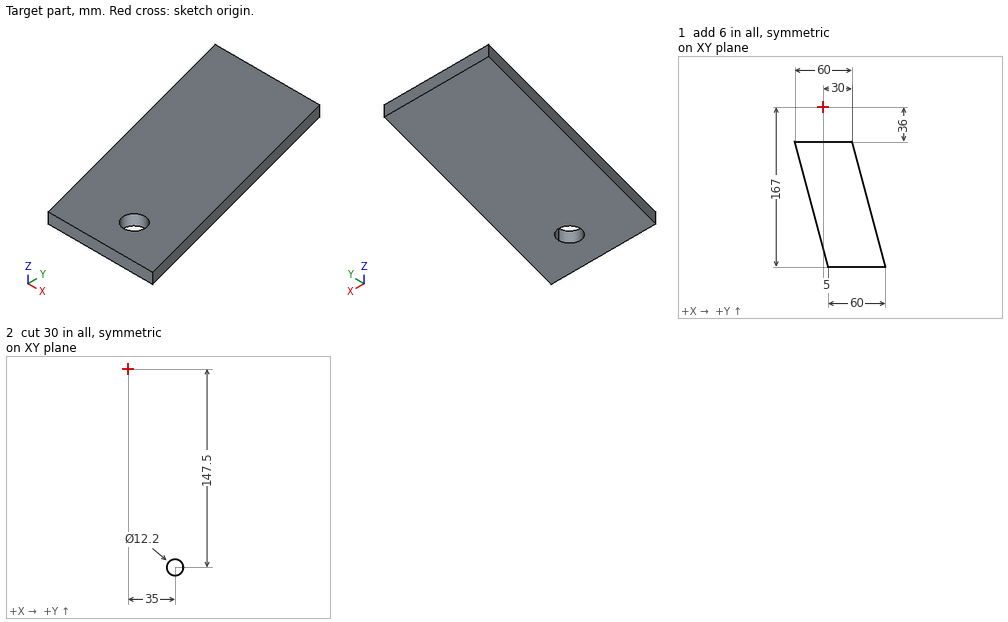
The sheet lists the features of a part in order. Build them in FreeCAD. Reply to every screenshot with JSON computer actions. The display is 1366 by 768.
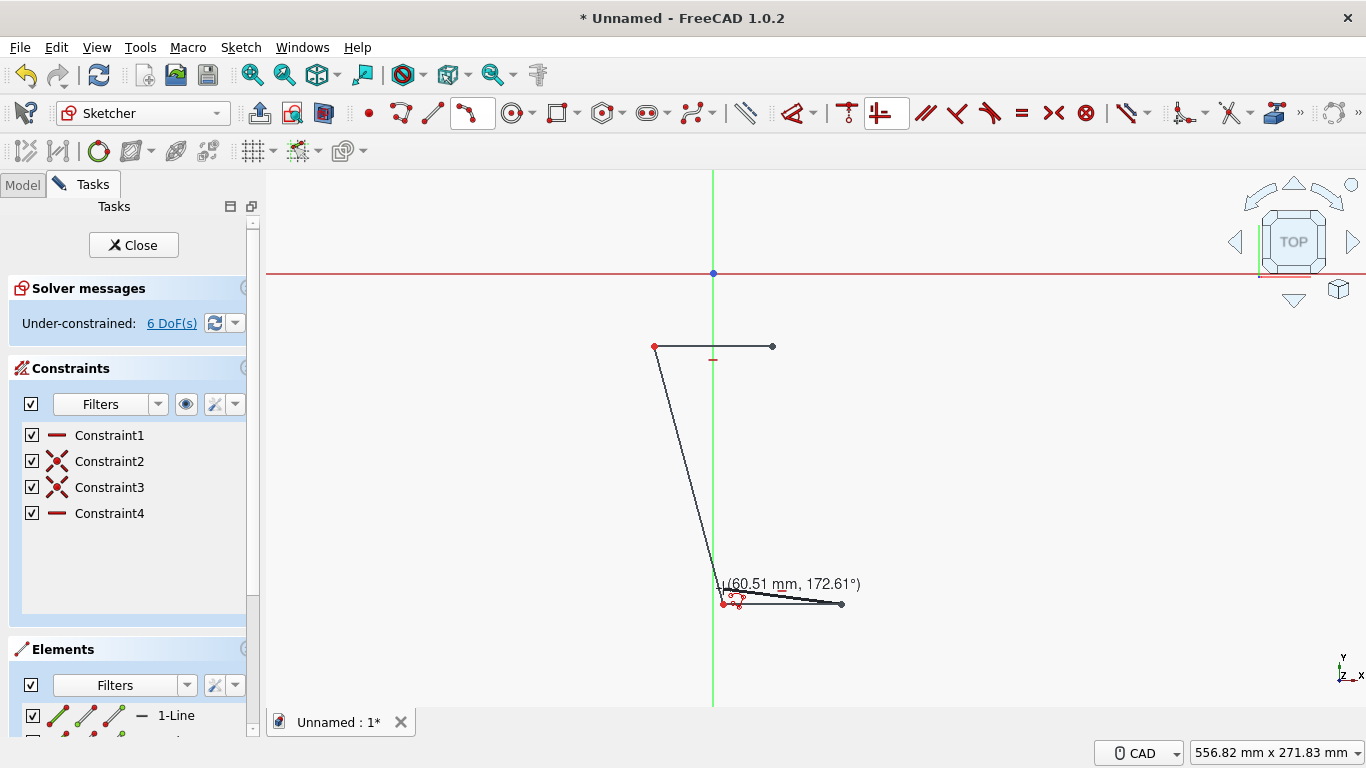
{"action": "left_click", "coordinate": [772, 346]}
{"action": "key", "text": "Escape"}
{"action": "key", "text": "Escape"}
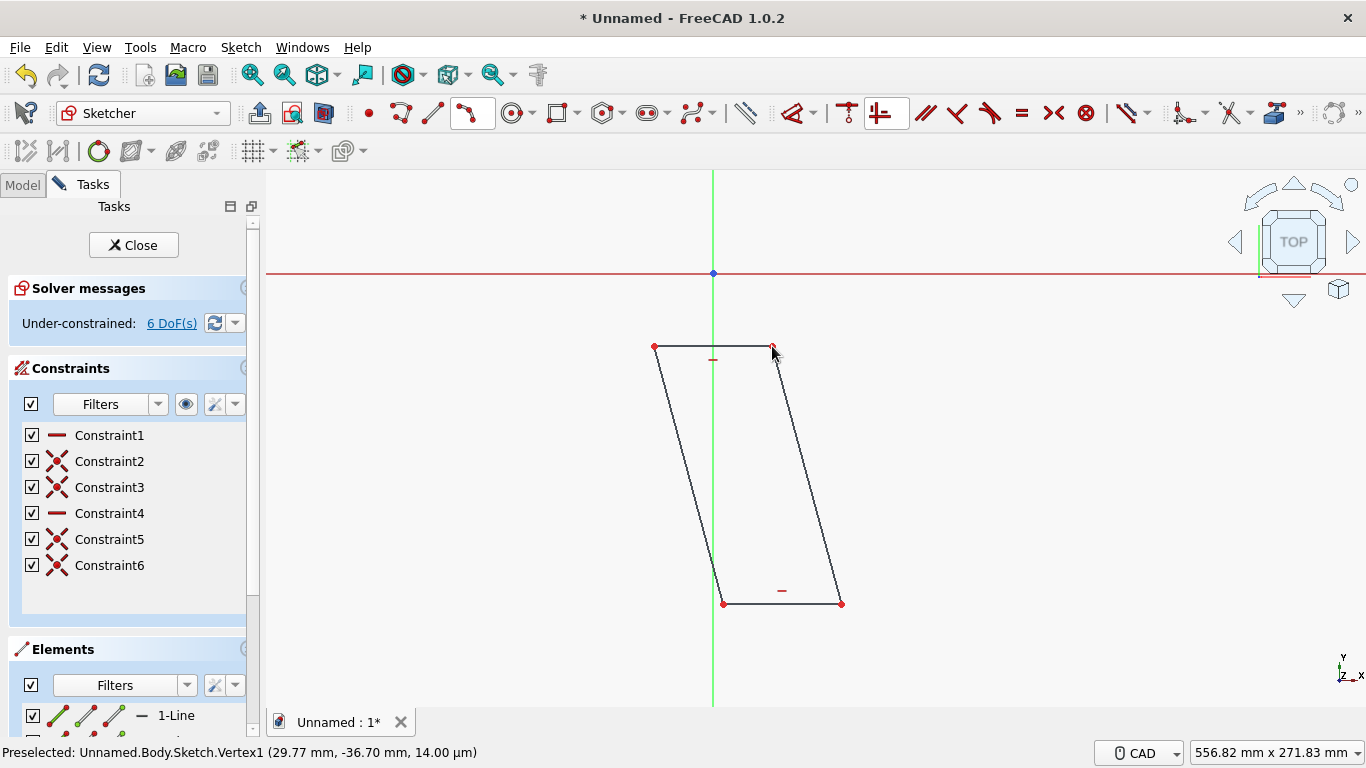
{"action": "left_click", "coordinate": [737, 346]}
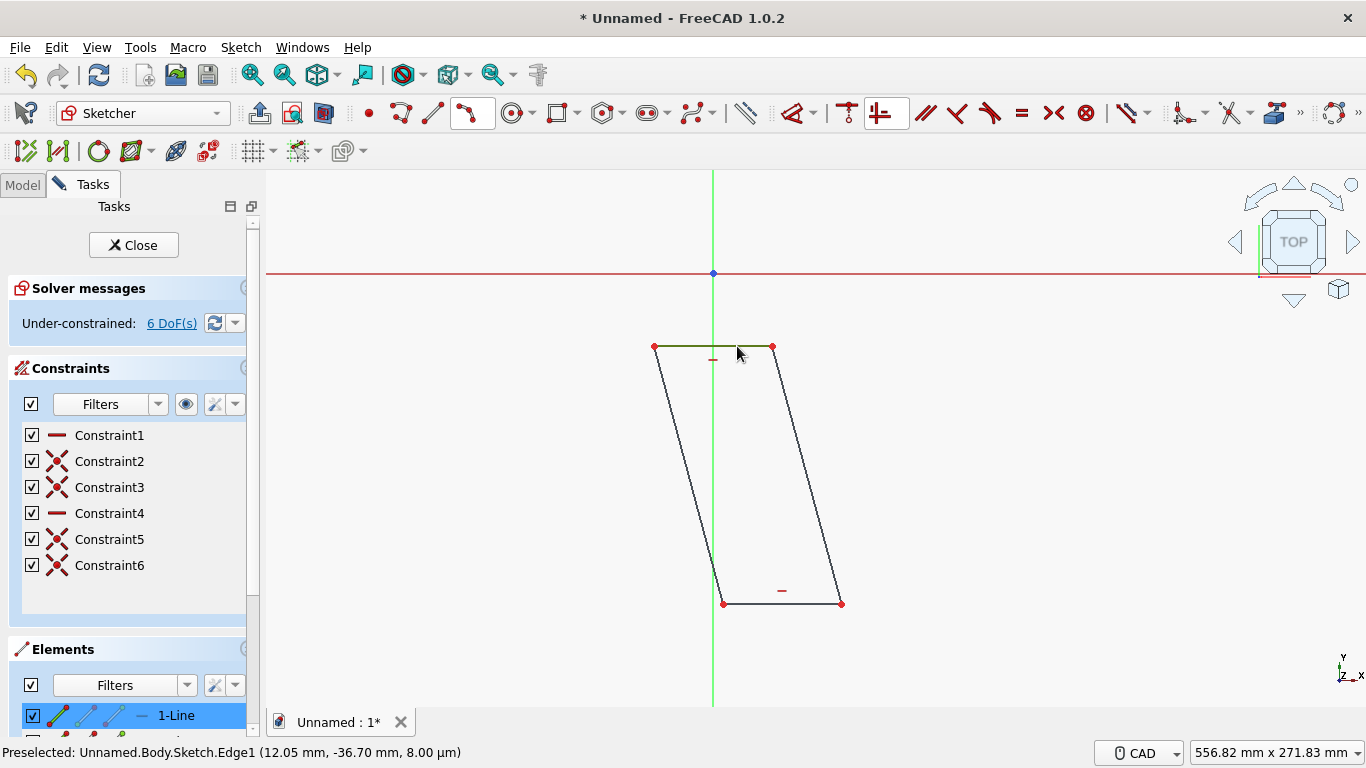
{"action": "left_click", "coordinate": [816, 114]}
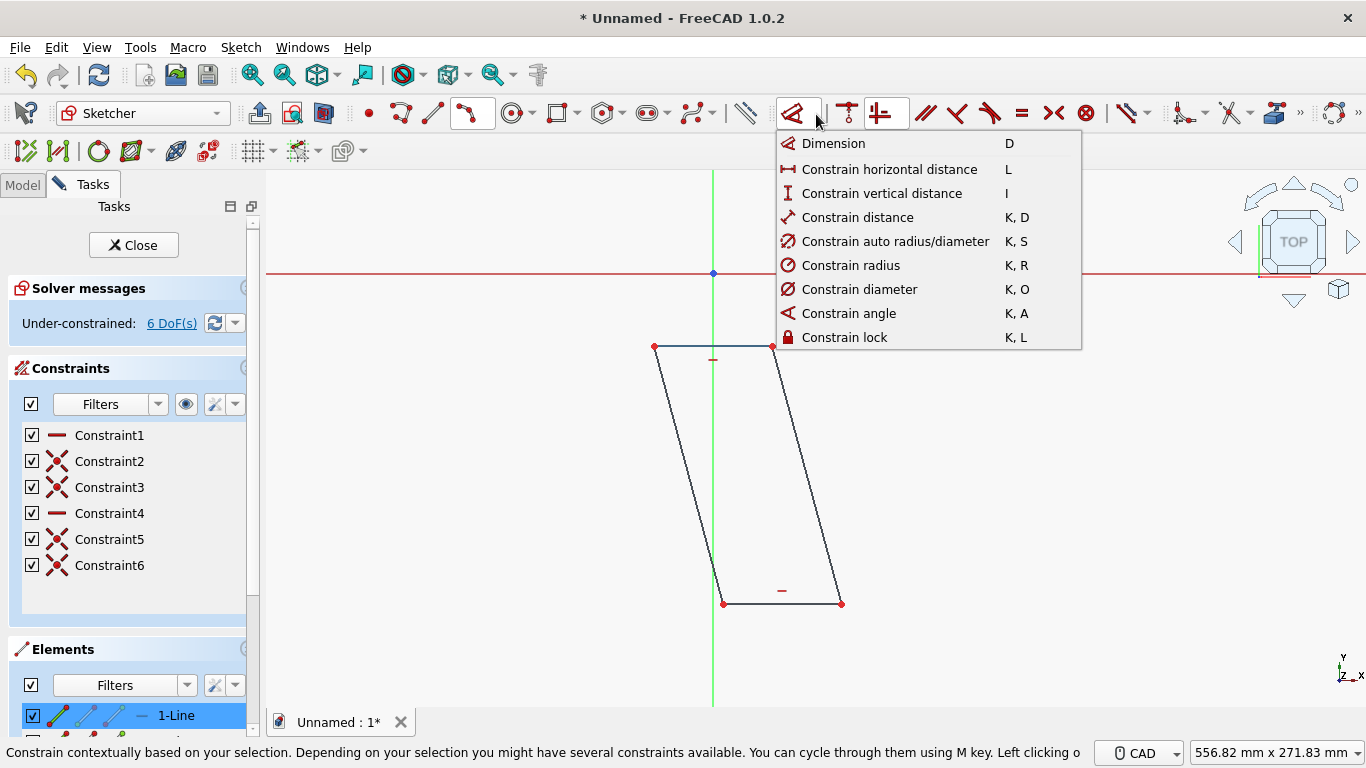
{"action": "left_click", "coordinate": [929, 169]}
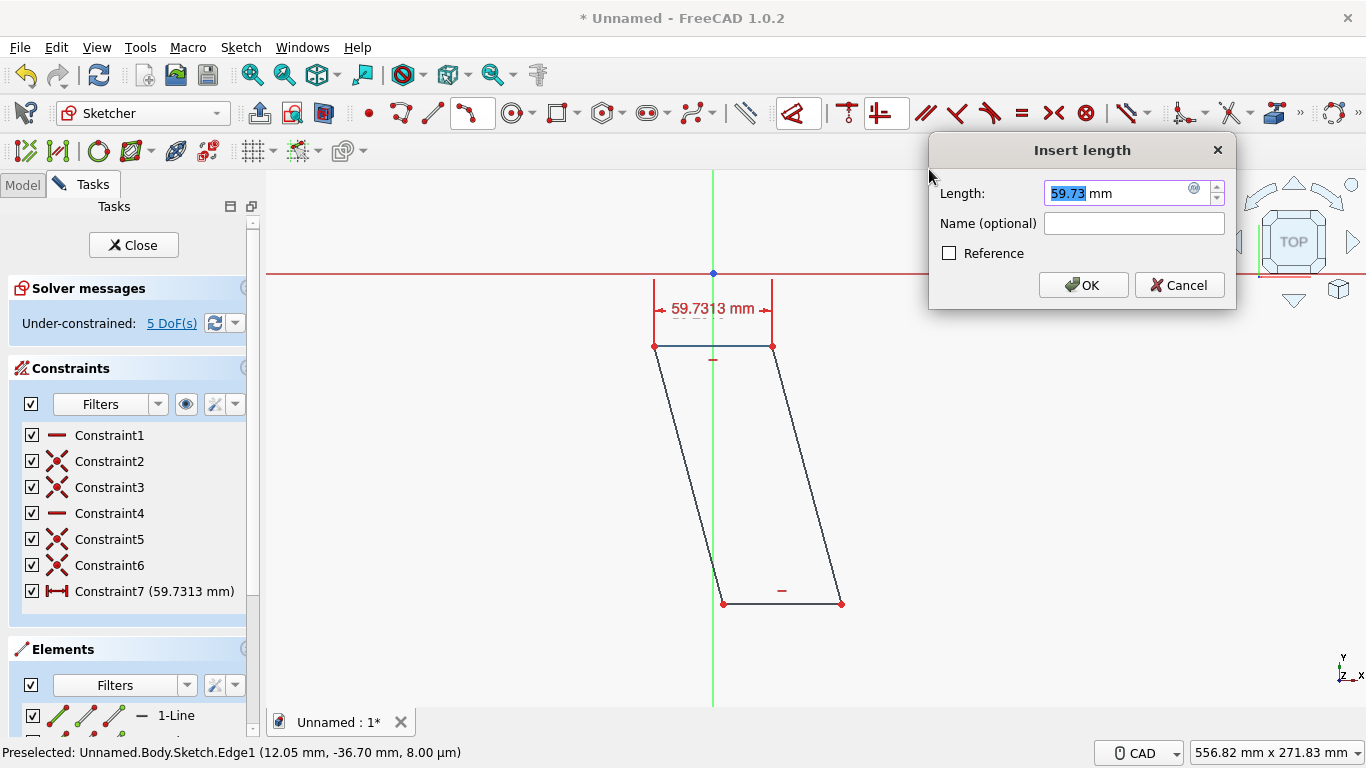
{"action": "type", "text": "60"}
{"action": "key", "text": "Return"}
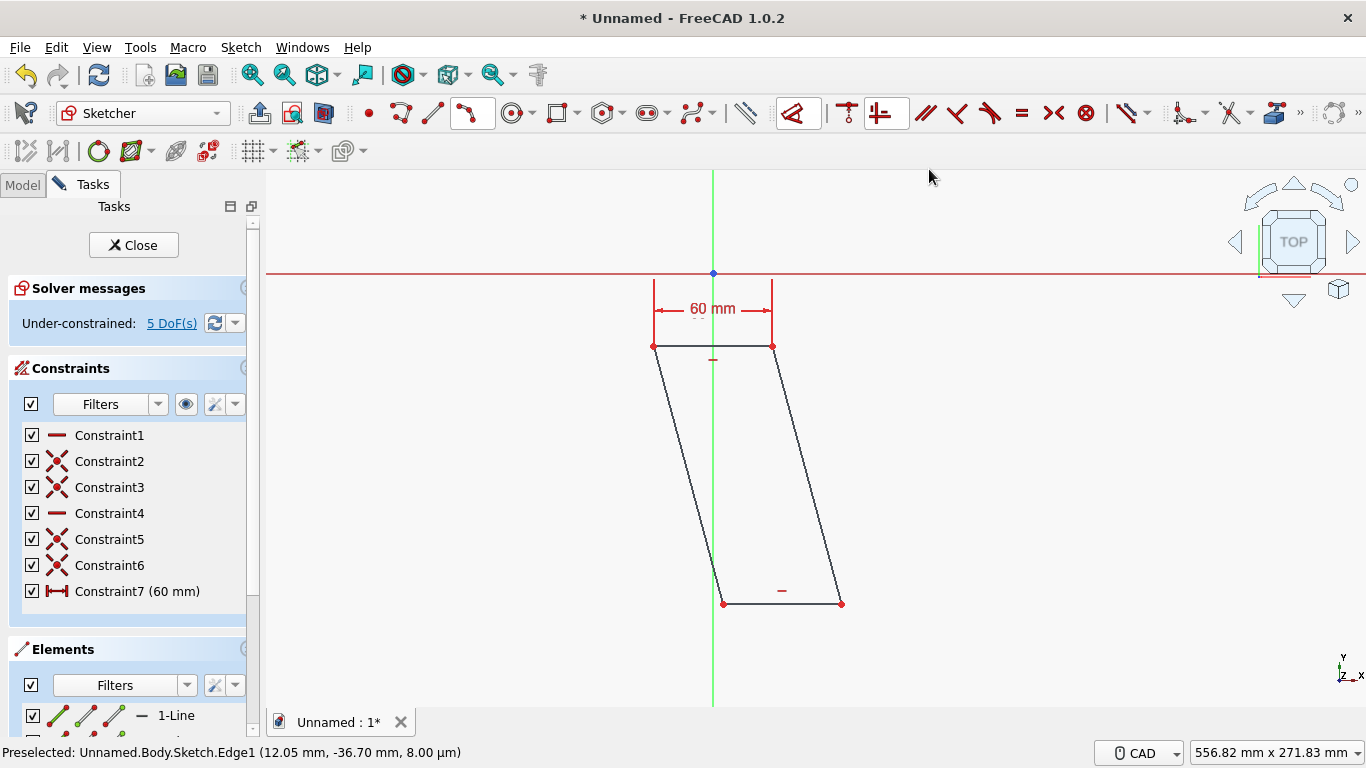
{"action": "left_click", "coordinate": [759, 604]}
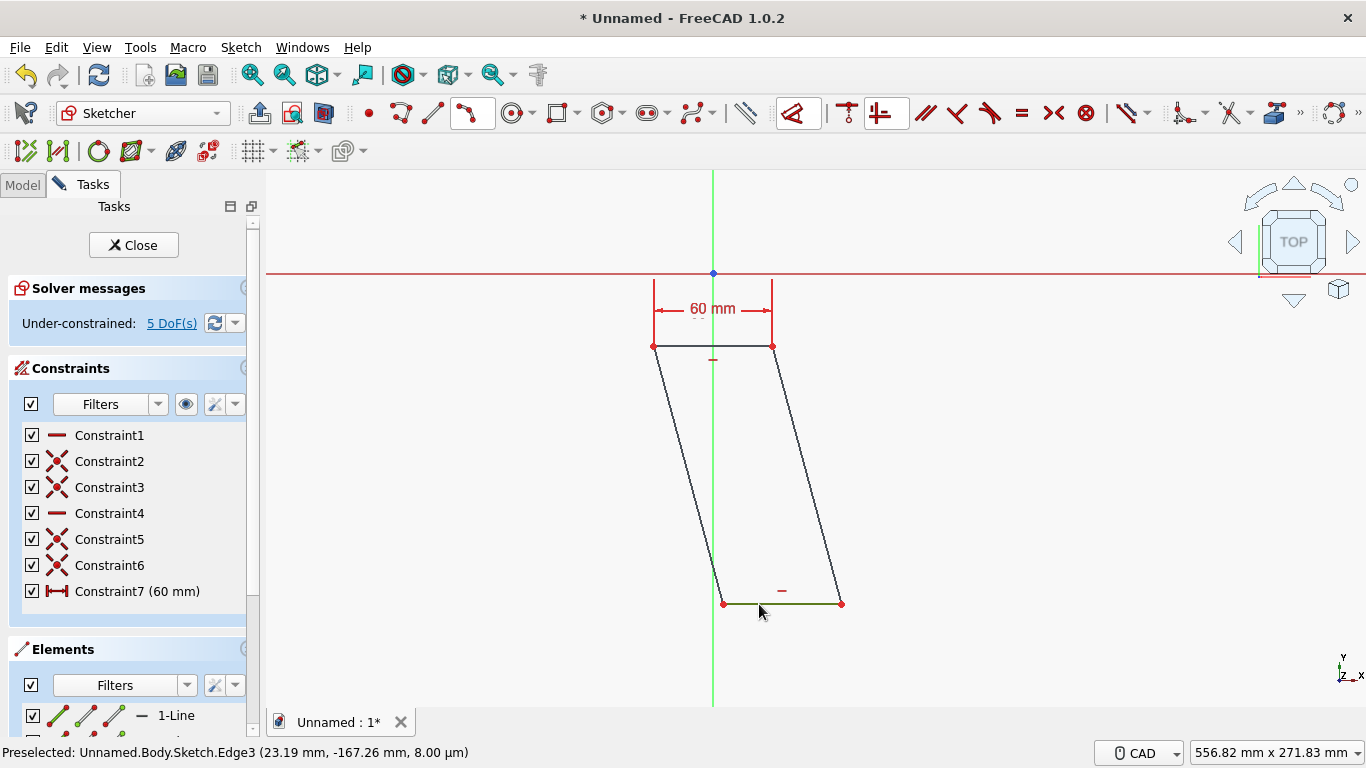
{"action": "key", "text": "l"}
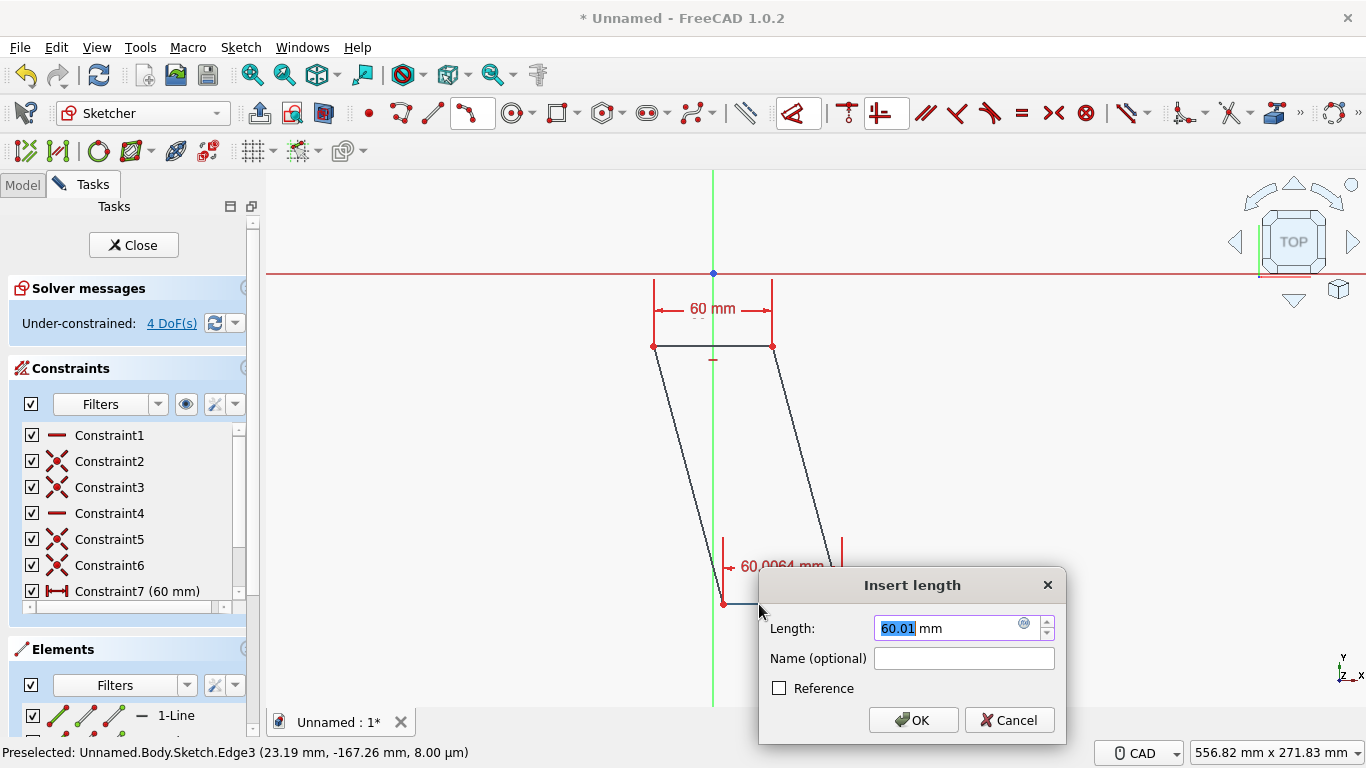
{"action": "type", "text": "60"}
{"action": "key", "text": "Return"}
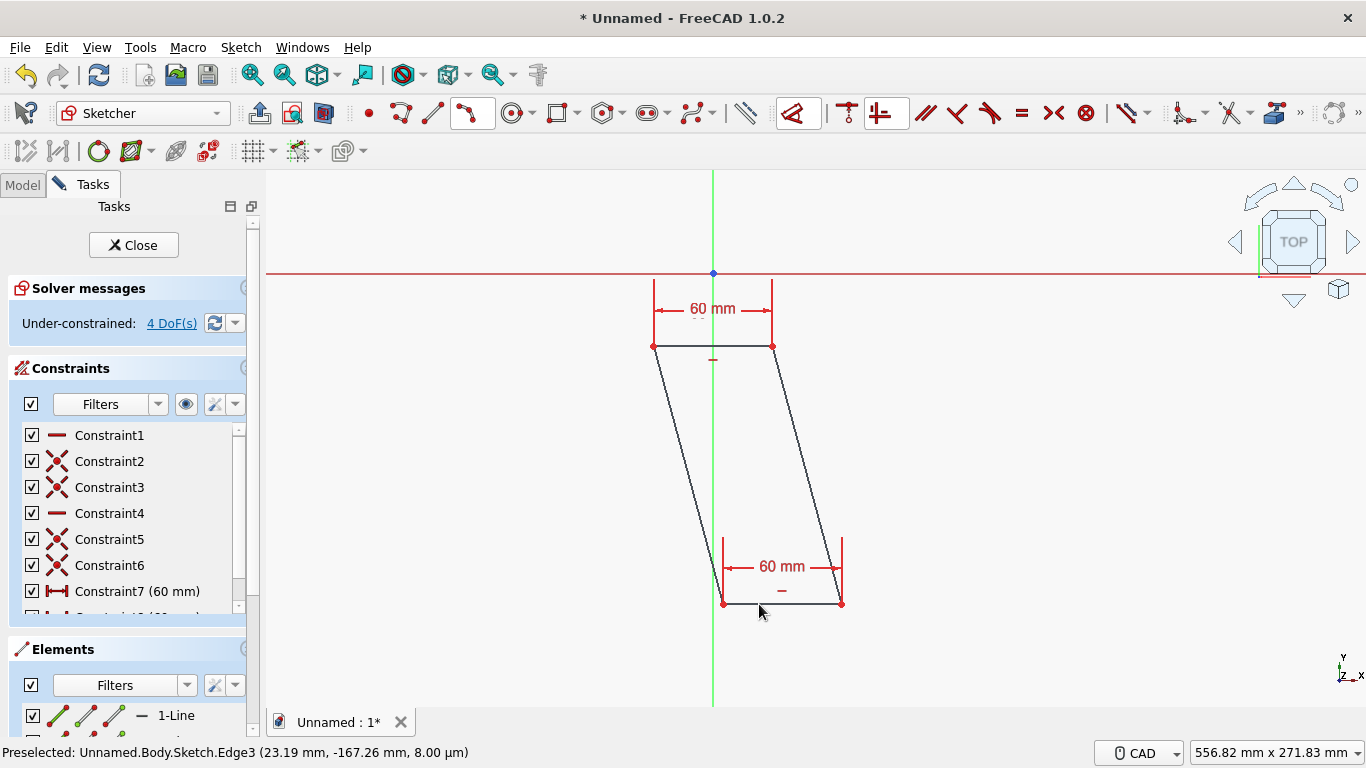
{"action": "scroll", "coordinate": [723, 604], "scroll_direction": "up", "scroll_amount": 7}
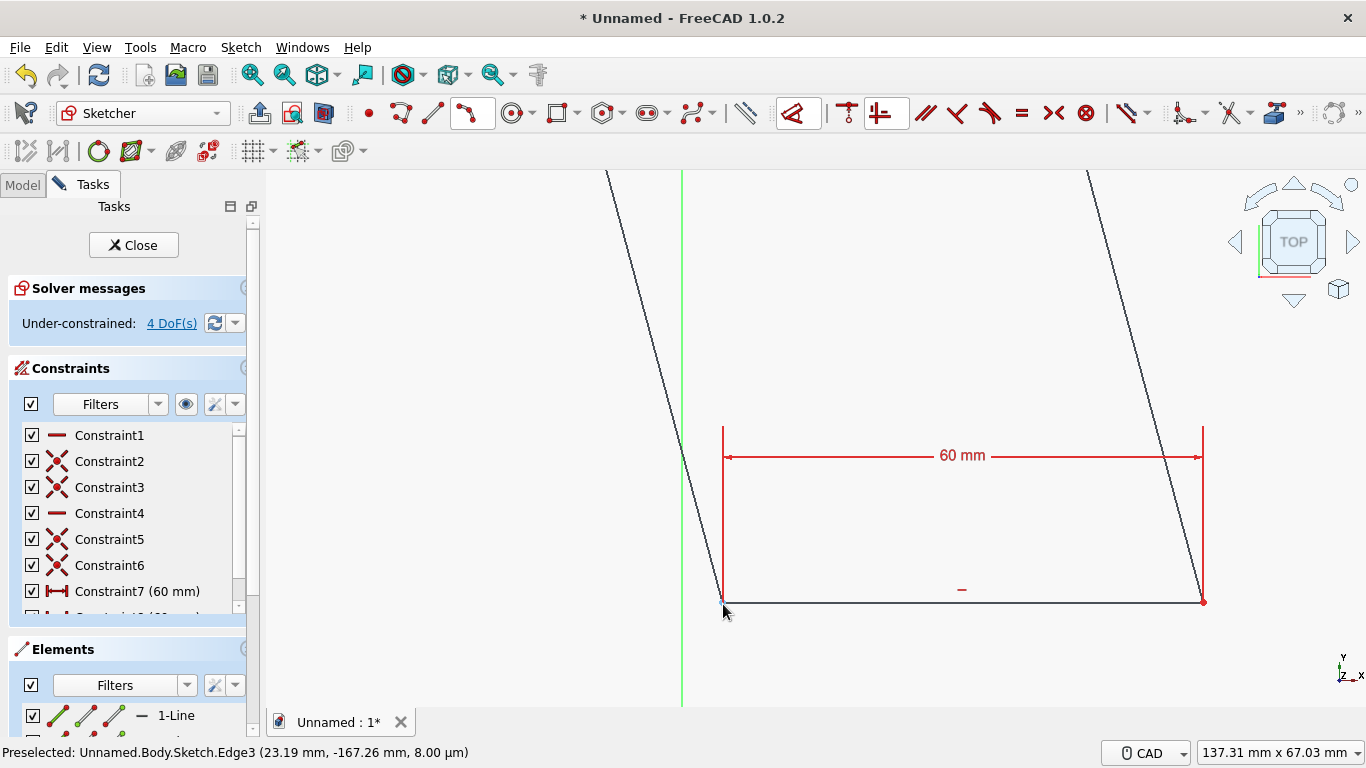
{"action": "left_click", "coordinate": [723, 603]}